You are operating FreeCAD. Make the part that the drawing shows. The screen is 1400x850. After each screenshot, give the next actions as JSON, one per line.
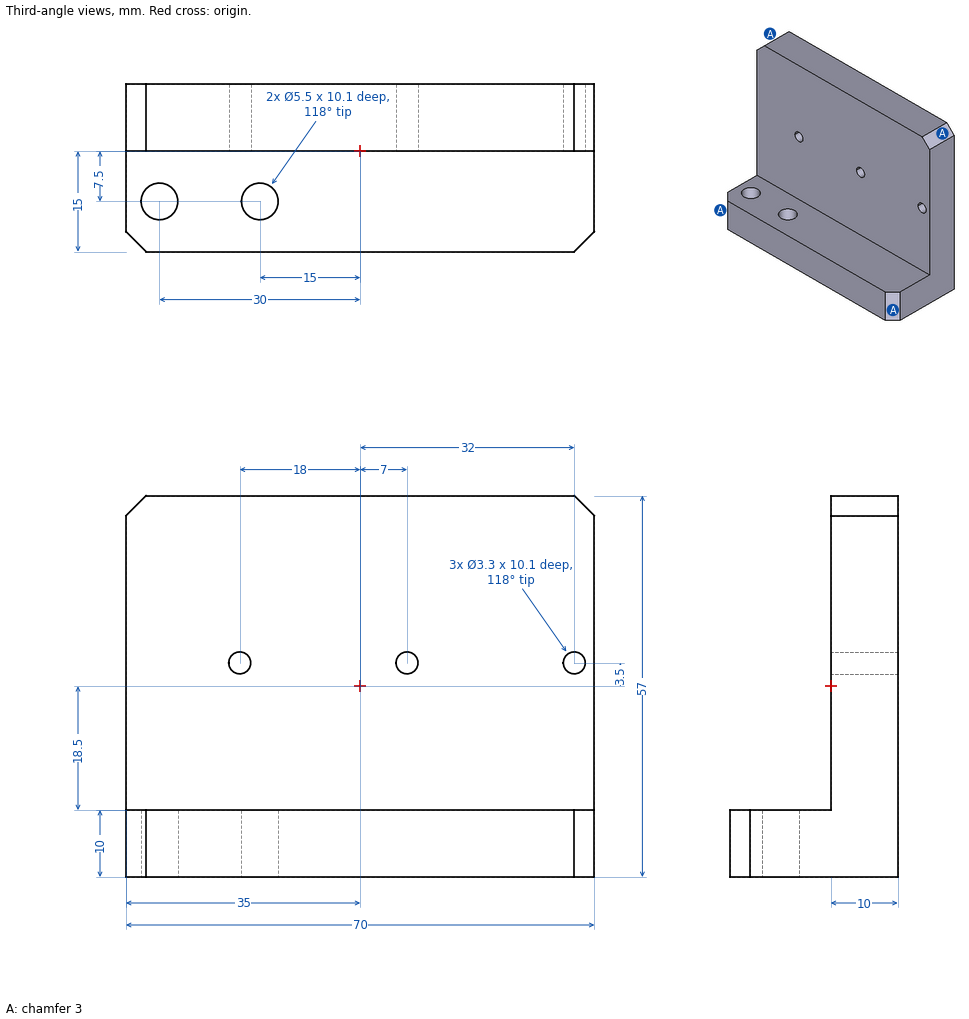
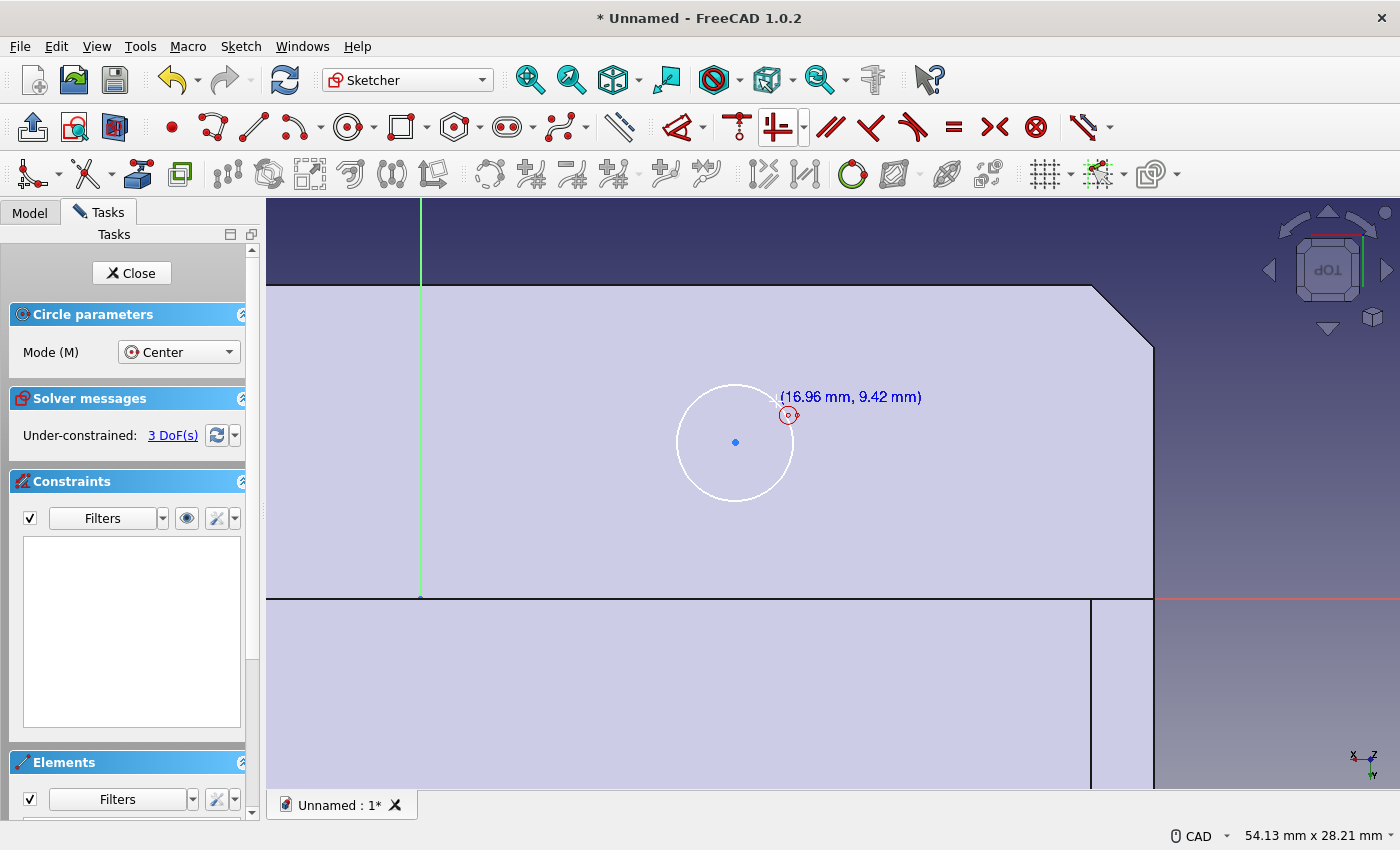
{"action": "left_click", "coordinate": [1049, 442]}
{"action": "left_click", "coordinate": [1090, 401]}
{"action": "key", "text": "Escape"}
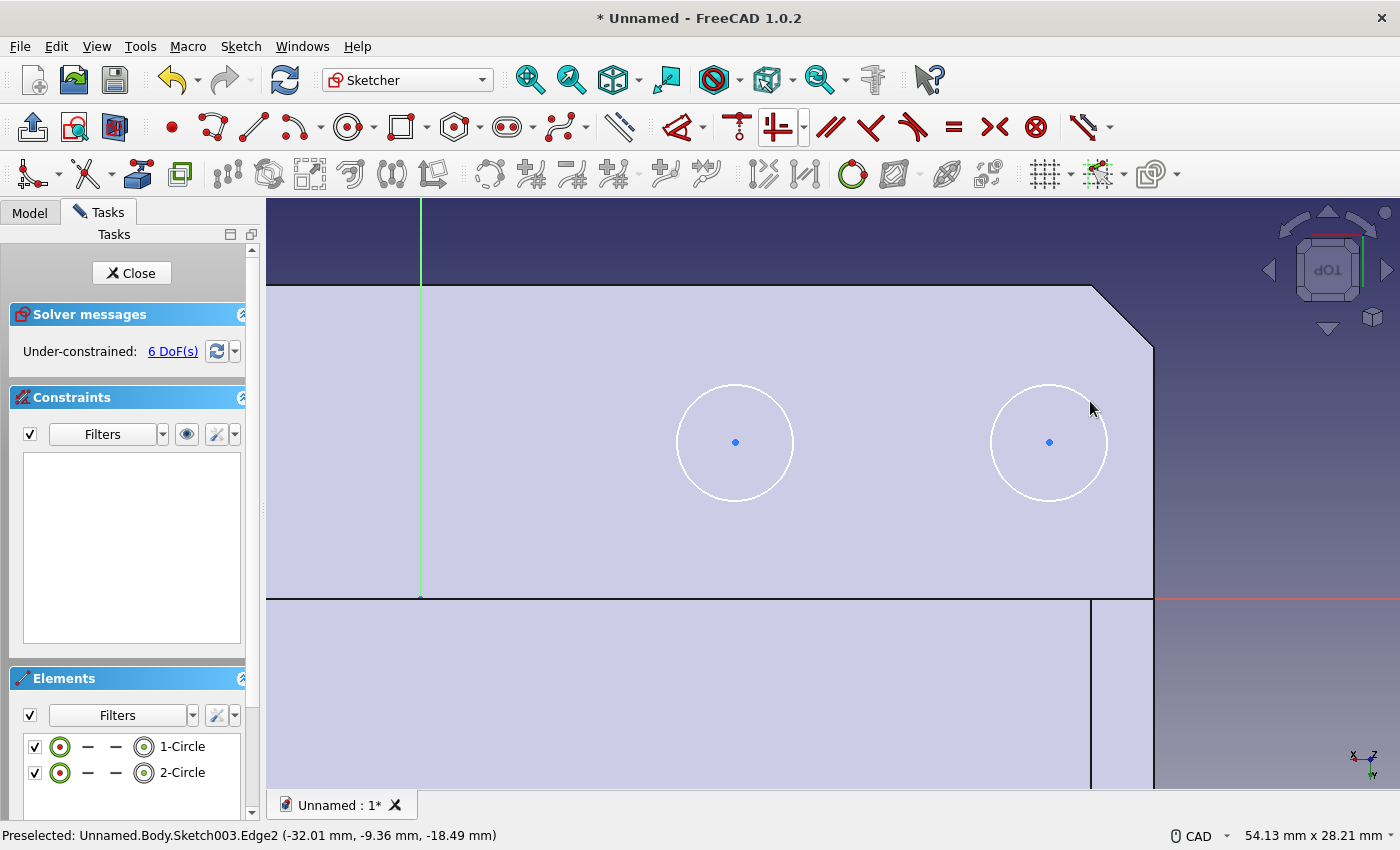
{"action": "left_click", "coordinate": [776, 402]}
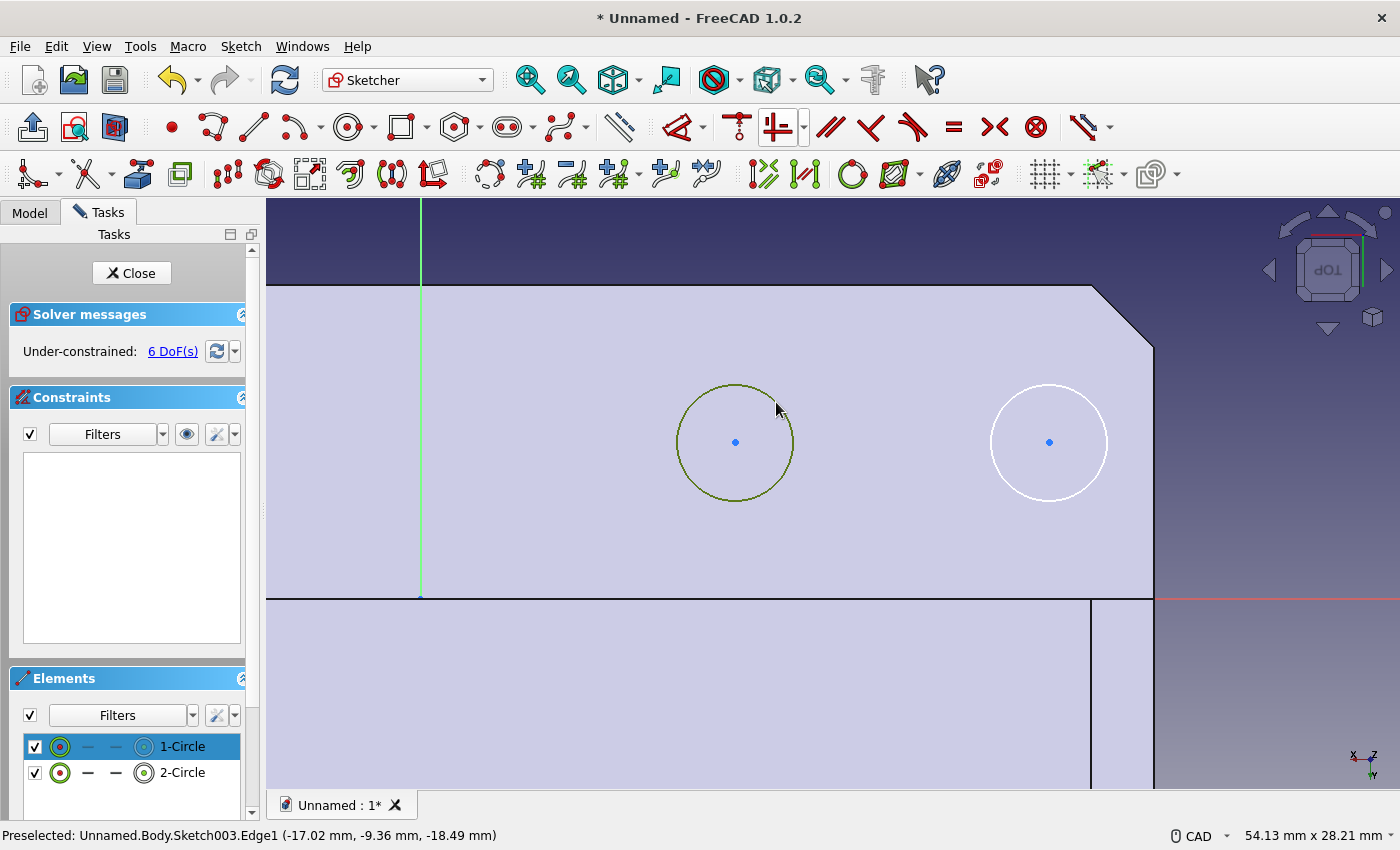
{"action": "left_click", "coordinate": [1090, 402]}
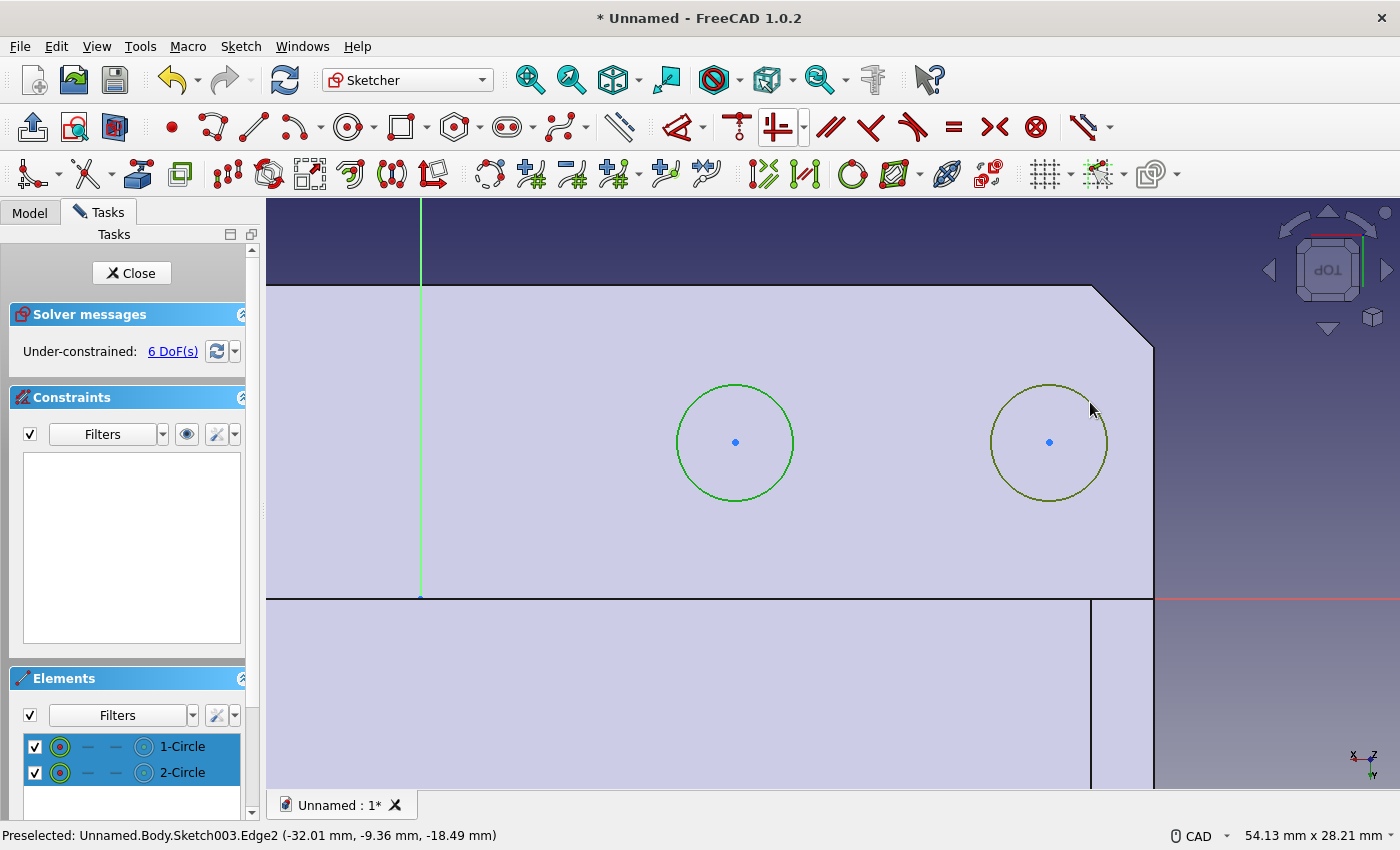
{"action": "left_click", "coordinate": [954, 128]}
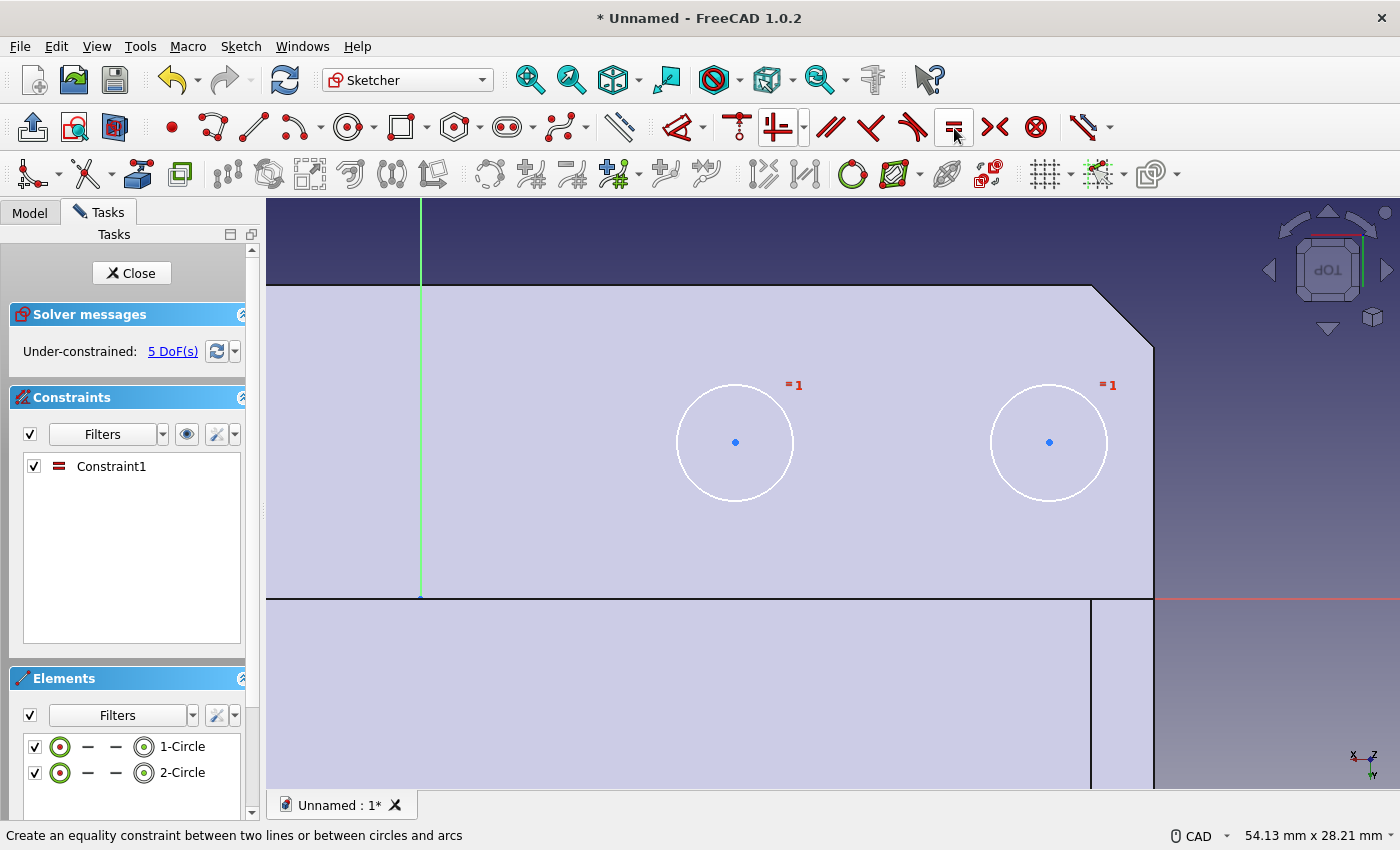
{"action": "left_click", "coordinate": [735, 443]}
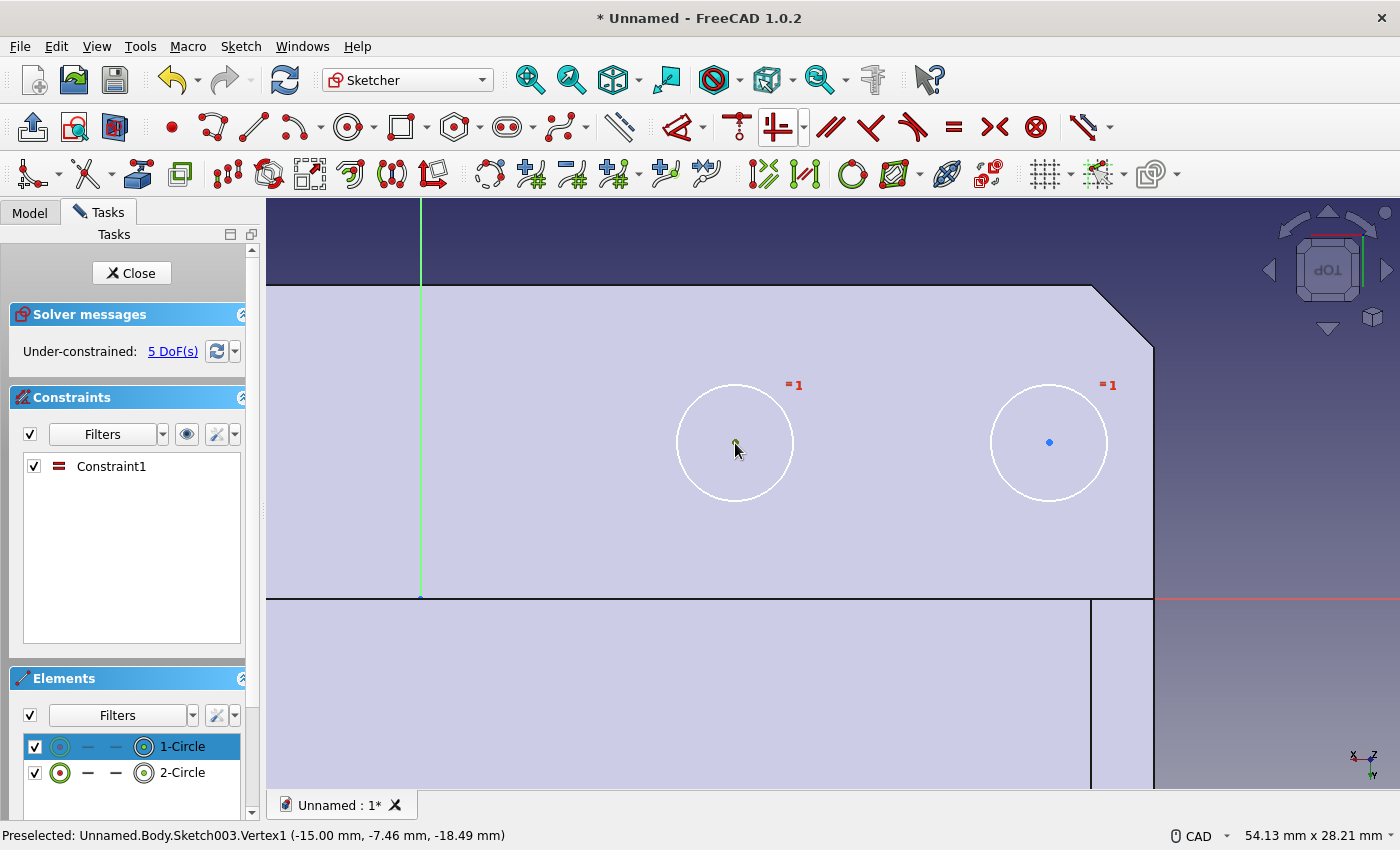
{"action": "left_click", "coordinate": [1049, 443]}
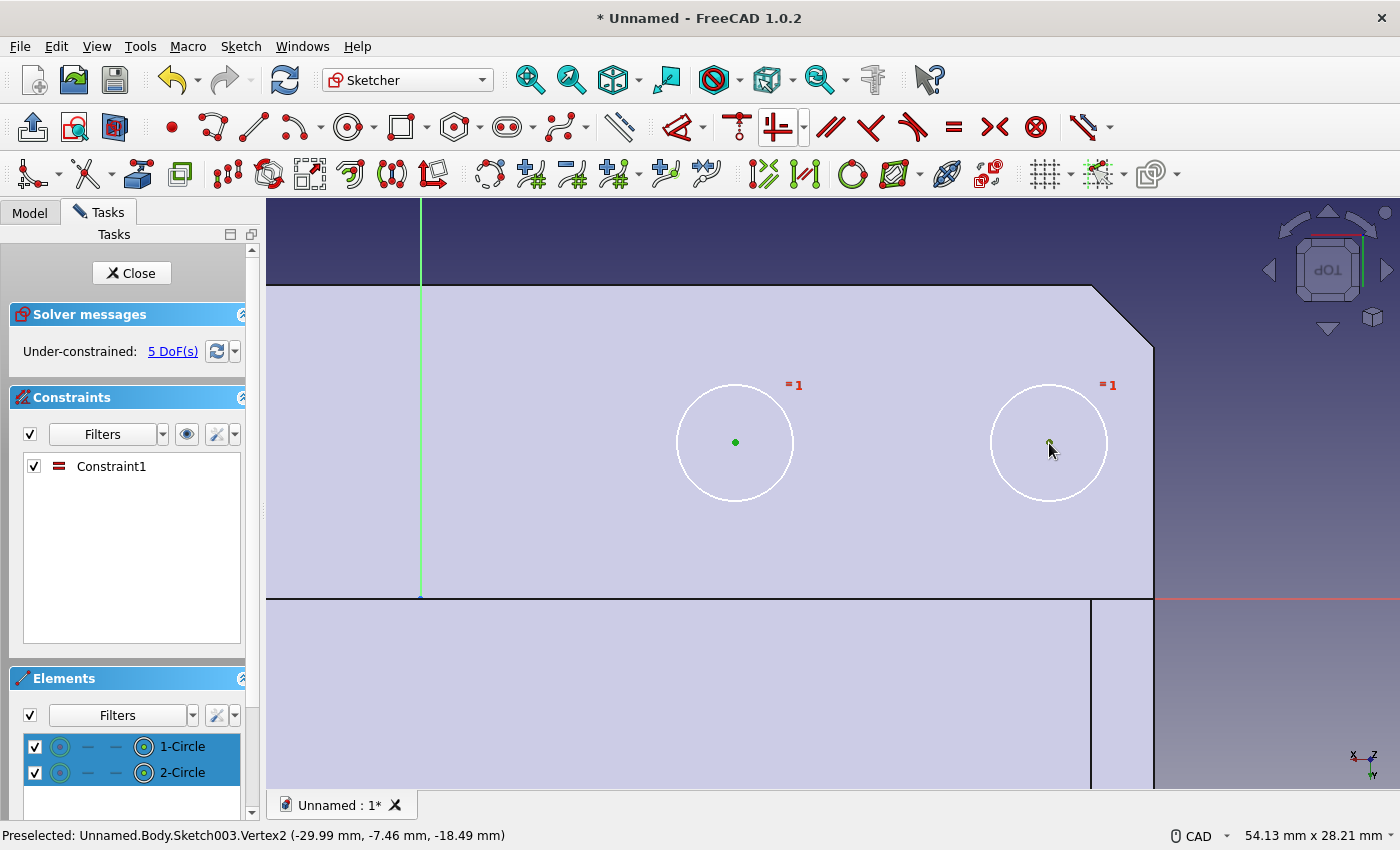
{"action": "key", "text": "h"}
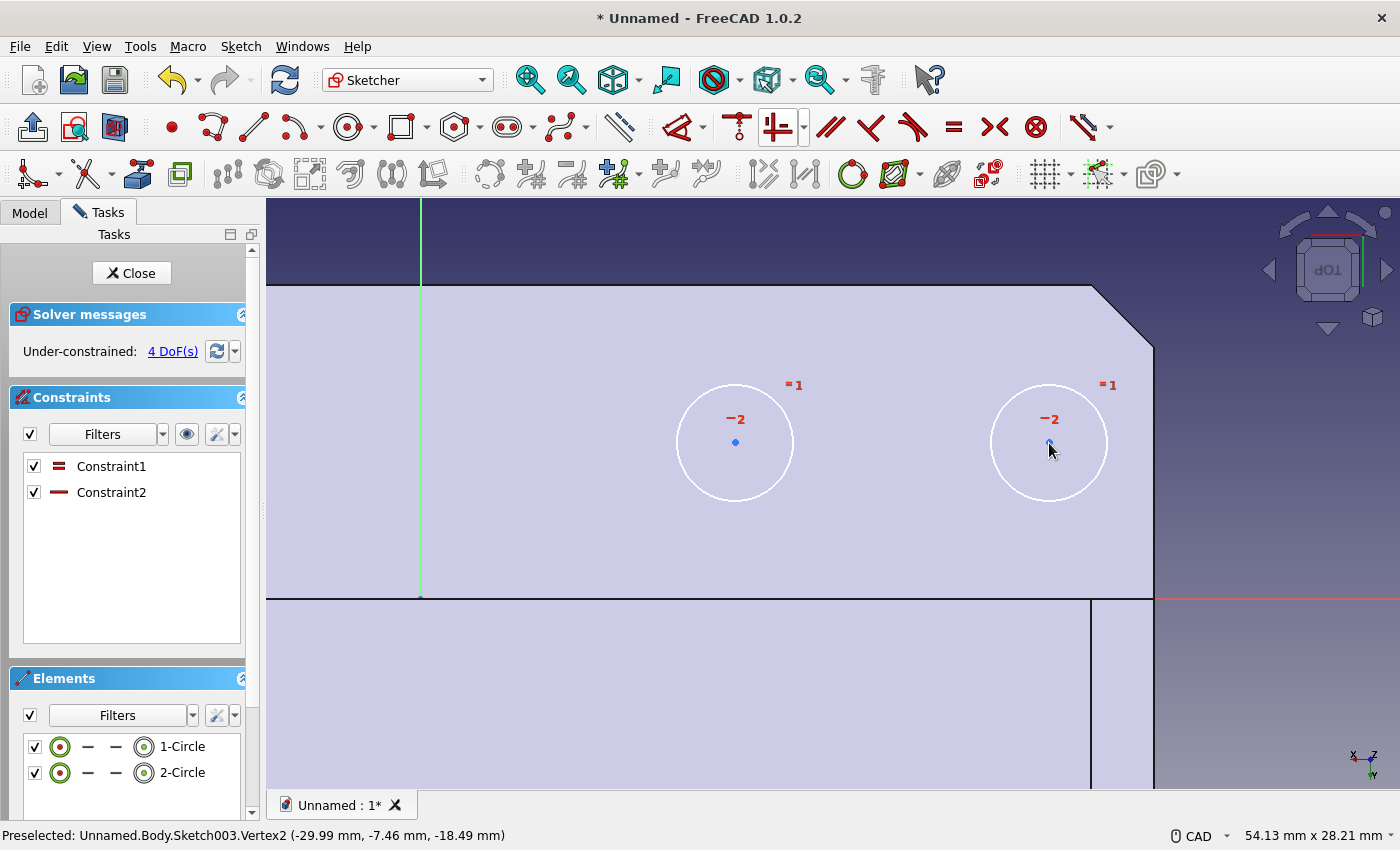
{"action": "left_click", "coordinate": [676, 128]}